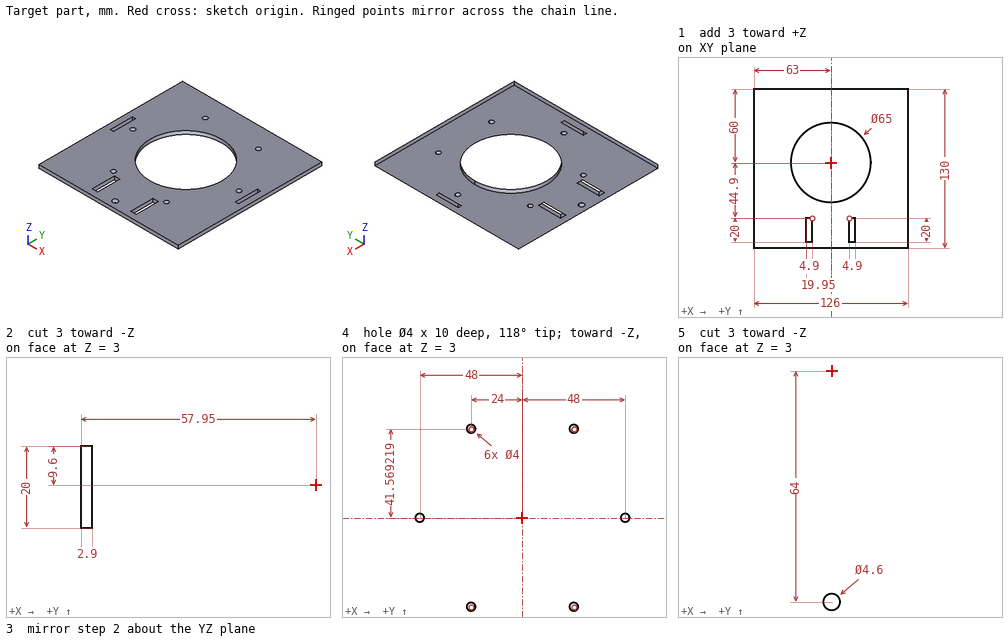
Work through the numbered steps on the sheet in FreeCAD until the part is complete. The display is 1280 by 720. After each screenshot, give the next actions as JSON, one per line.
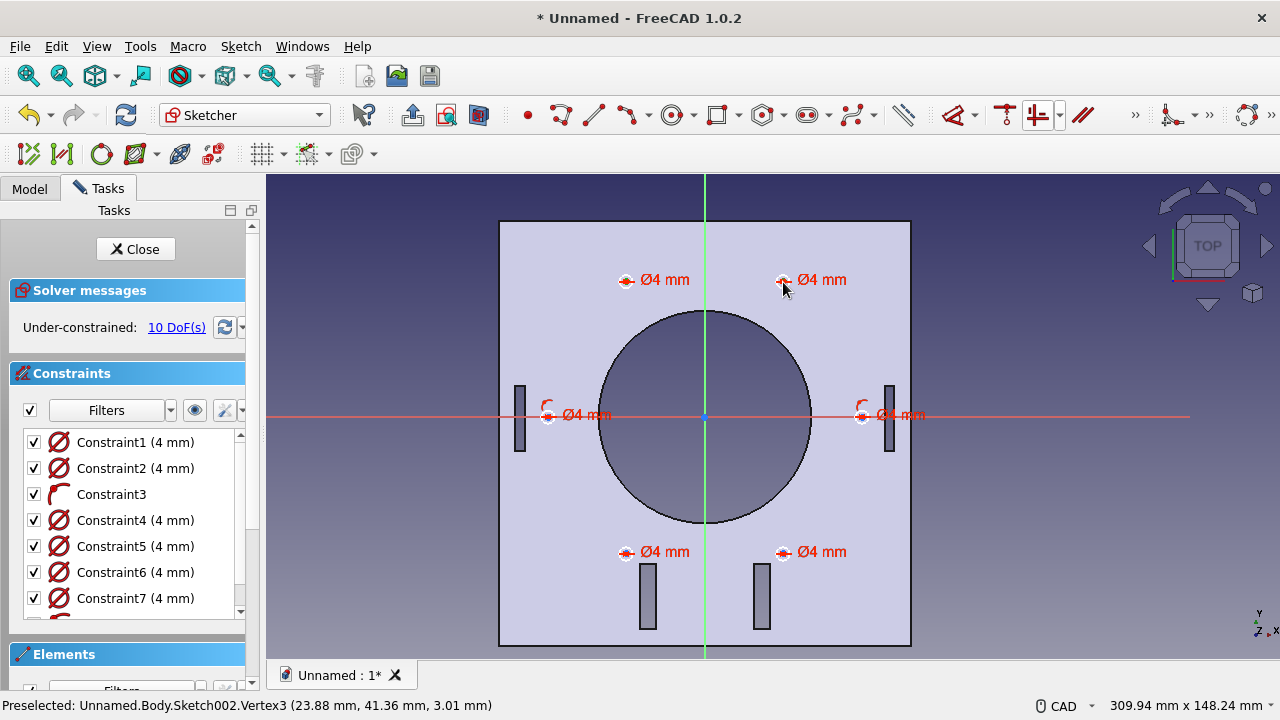
{"action": "left_click", "coordinate": [705, 600]}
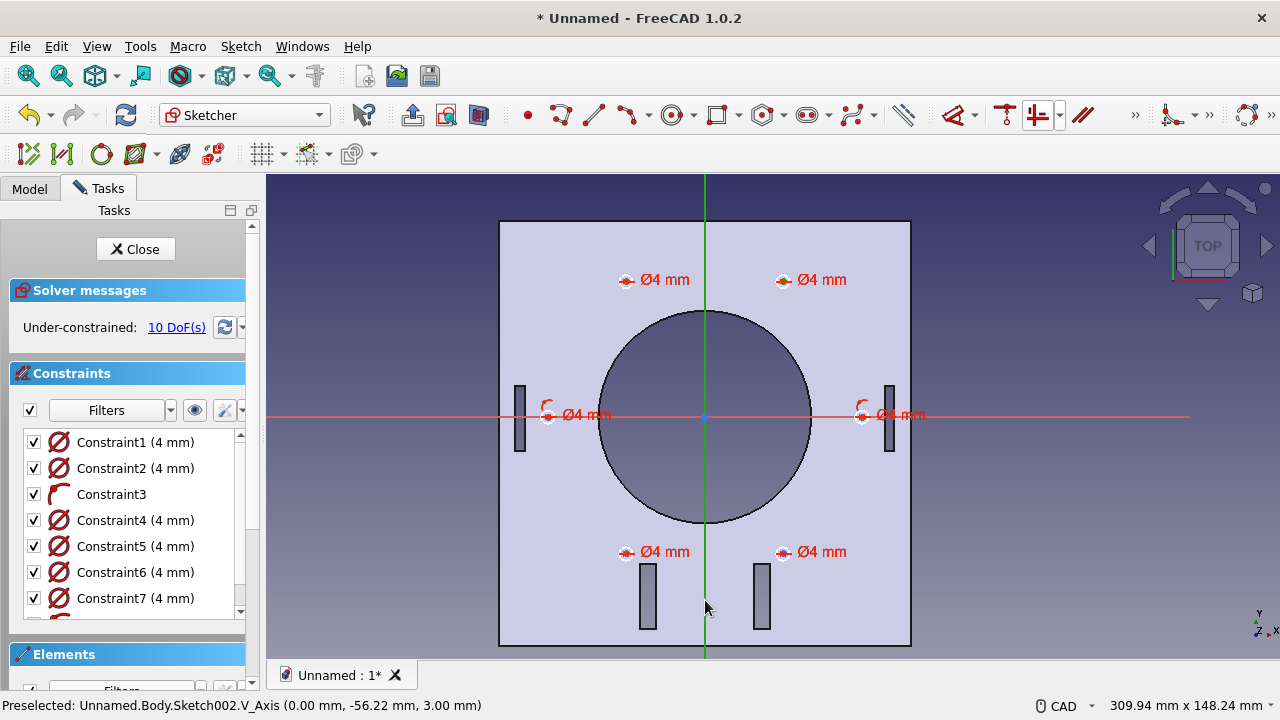
{"action": "key", "text": "s"}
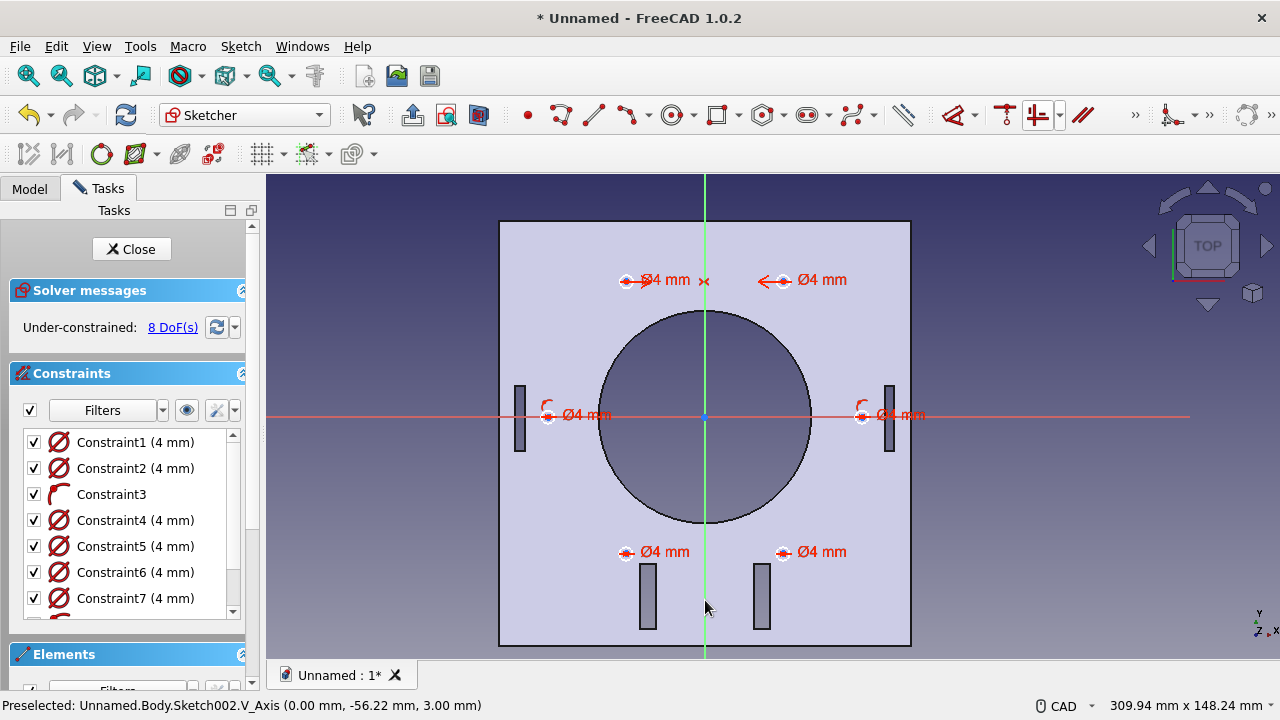
{"action": "left_click", "coordinate": [783, 282]}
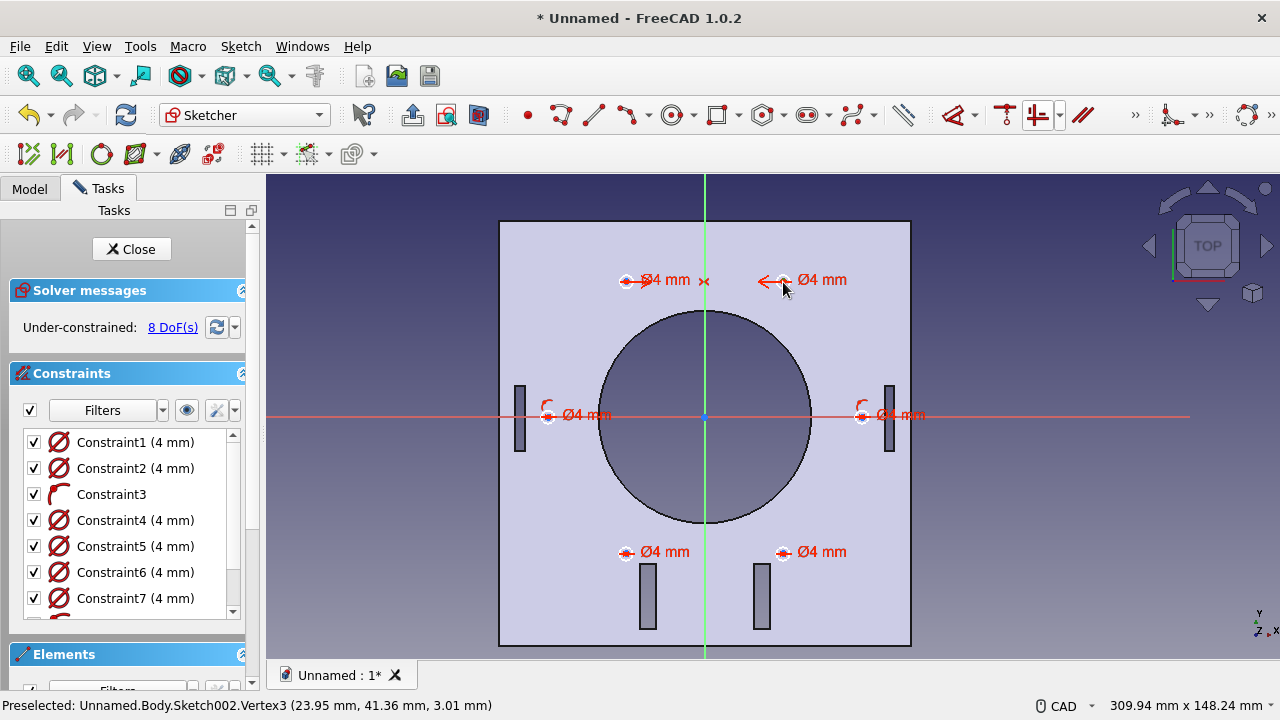
{"action": "left_click", "coordinate": [783, 554]}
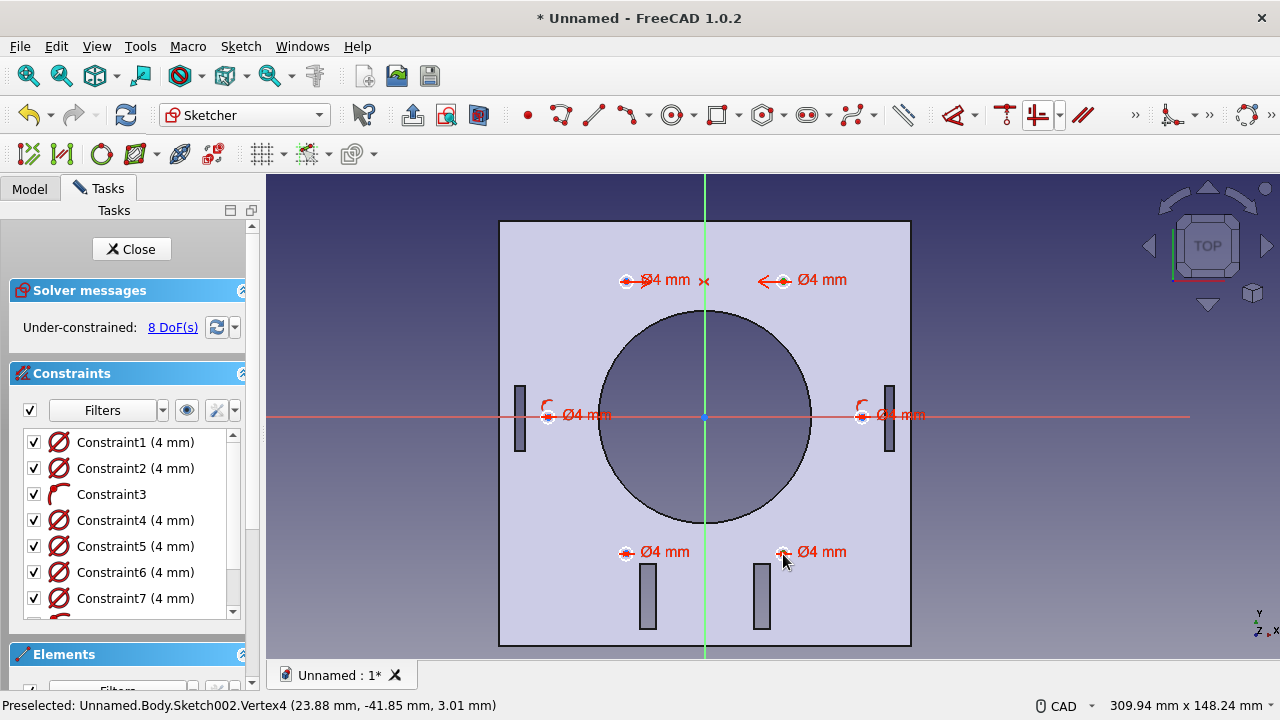
{"action": "left_click", "coordinate": [353, 417]}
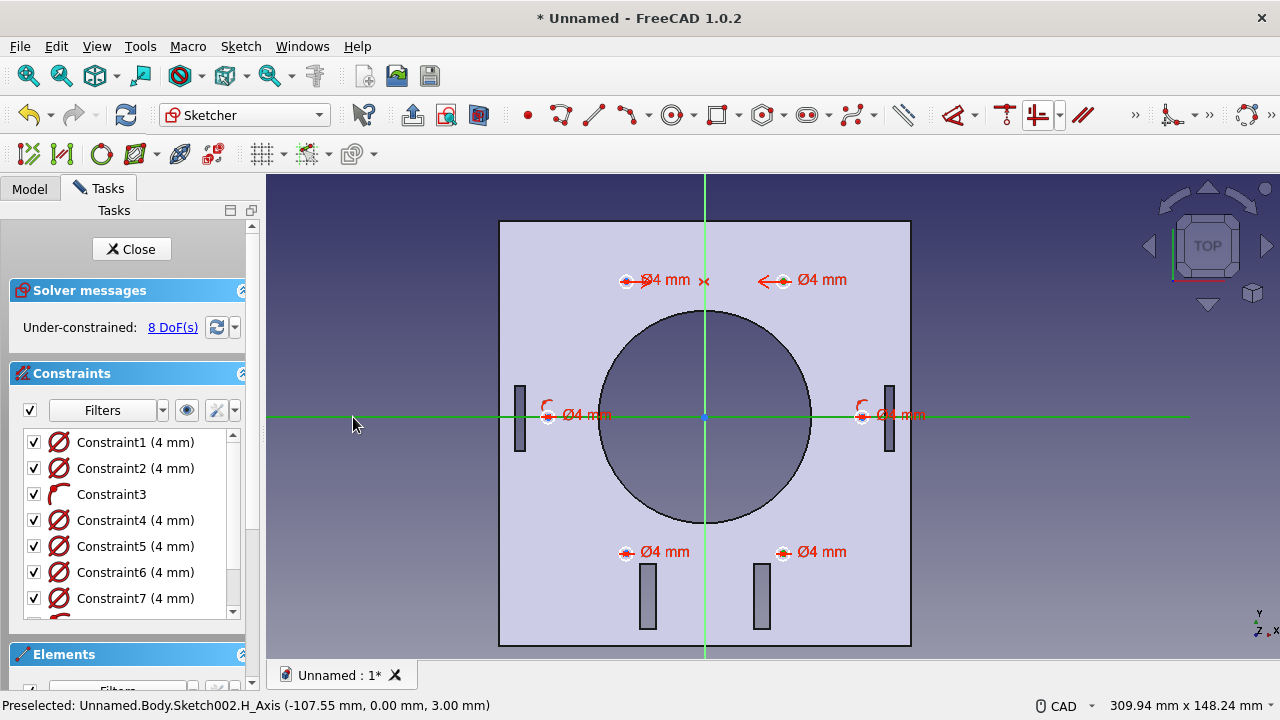
{"action": "key", "text": "s"}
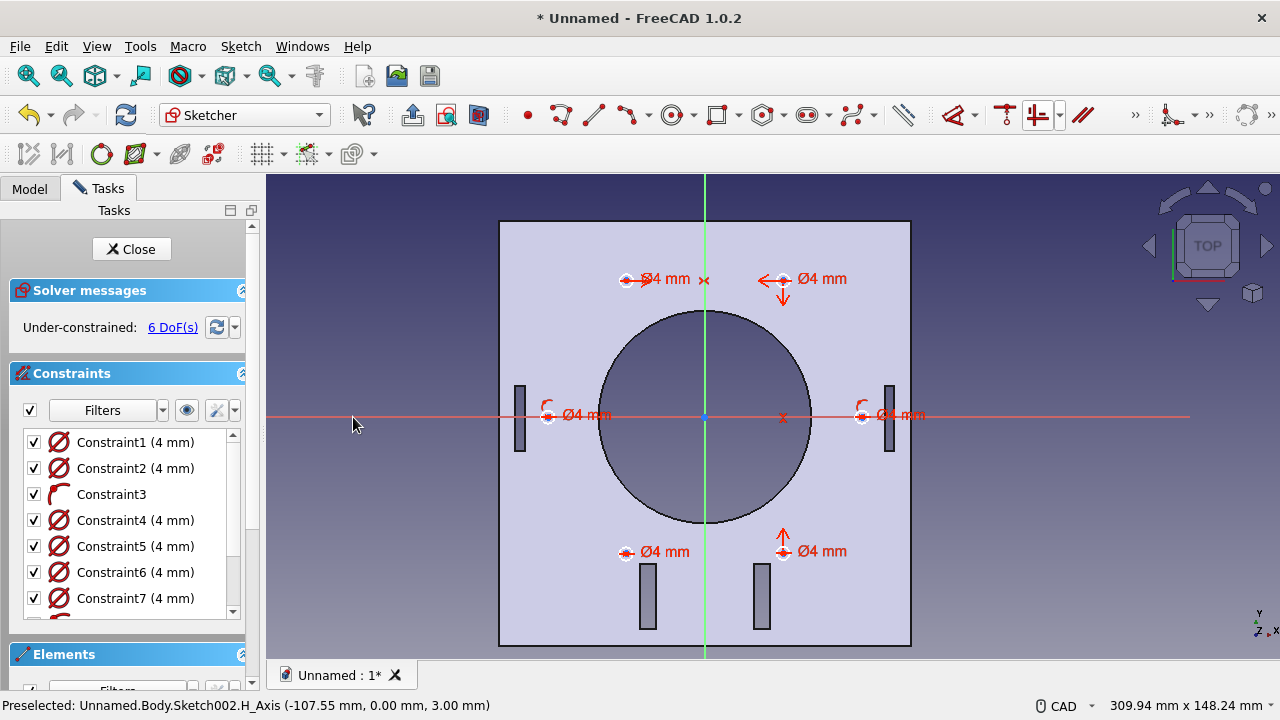
{"action": "left_click", "coordinate": [627, 281]}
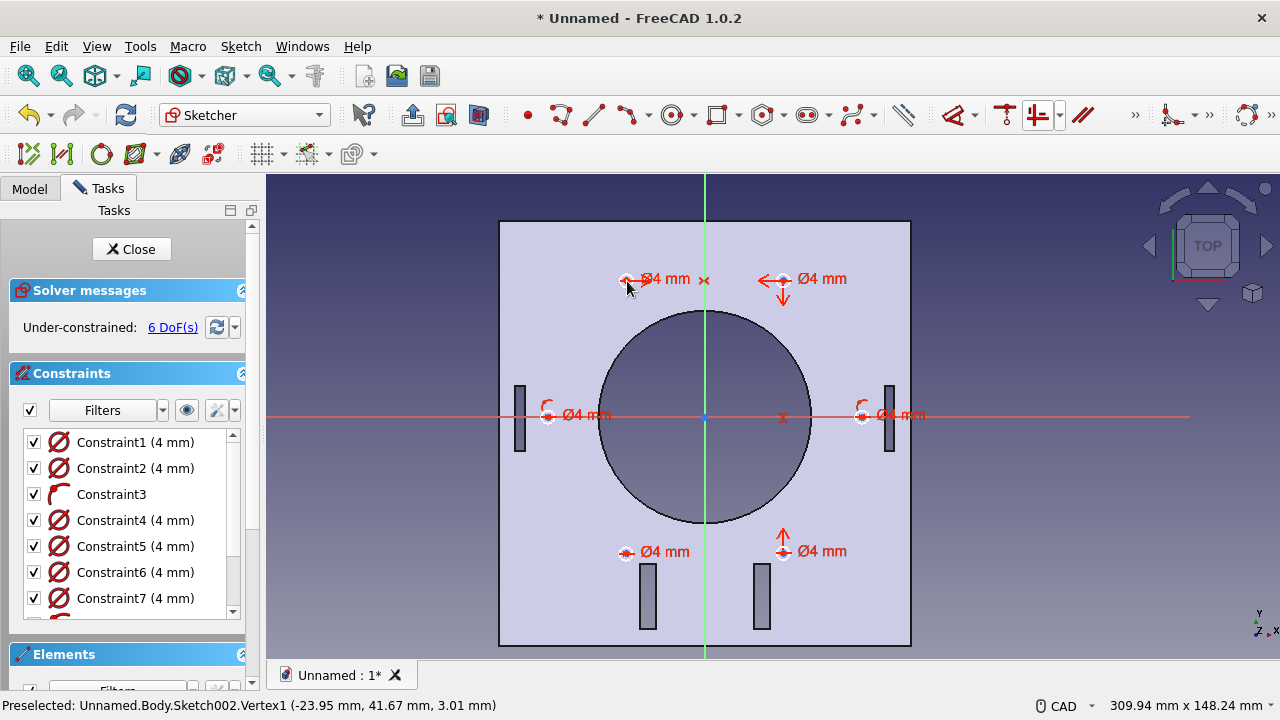
{"action": "left_click", "coordinate": [626, 554]}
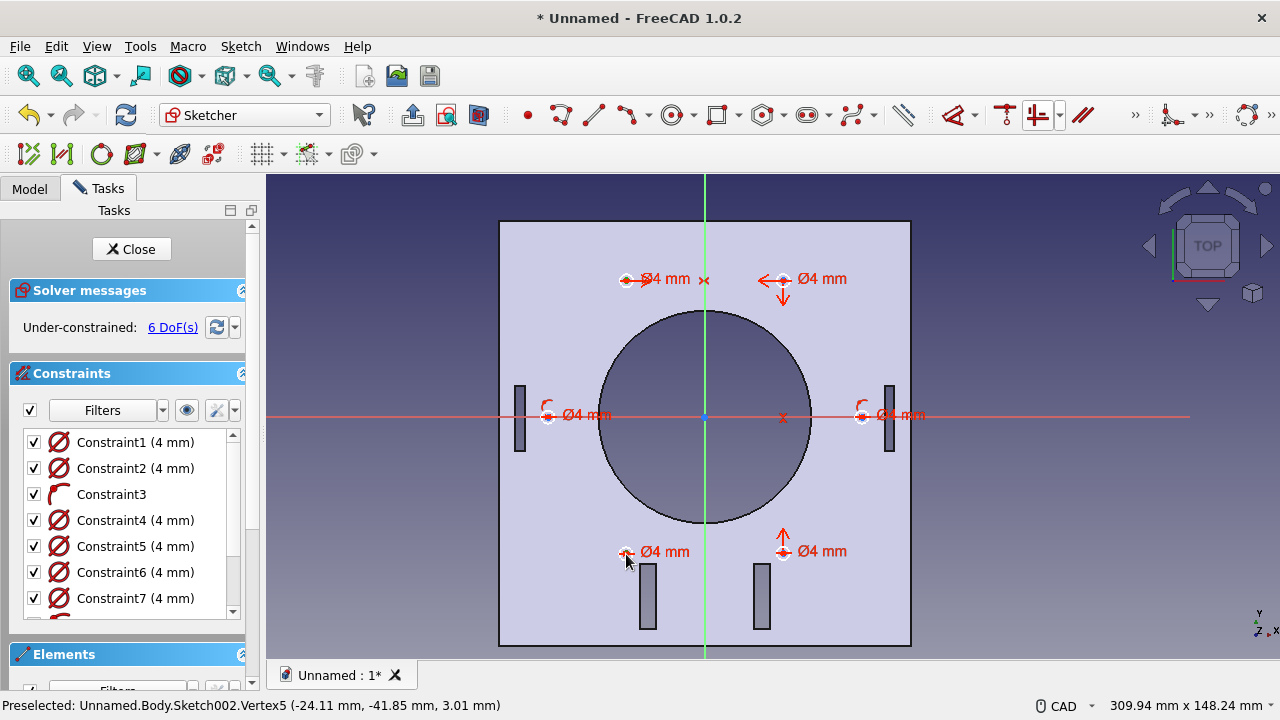
{"action": "left_click", "coordinate": [353, 417]}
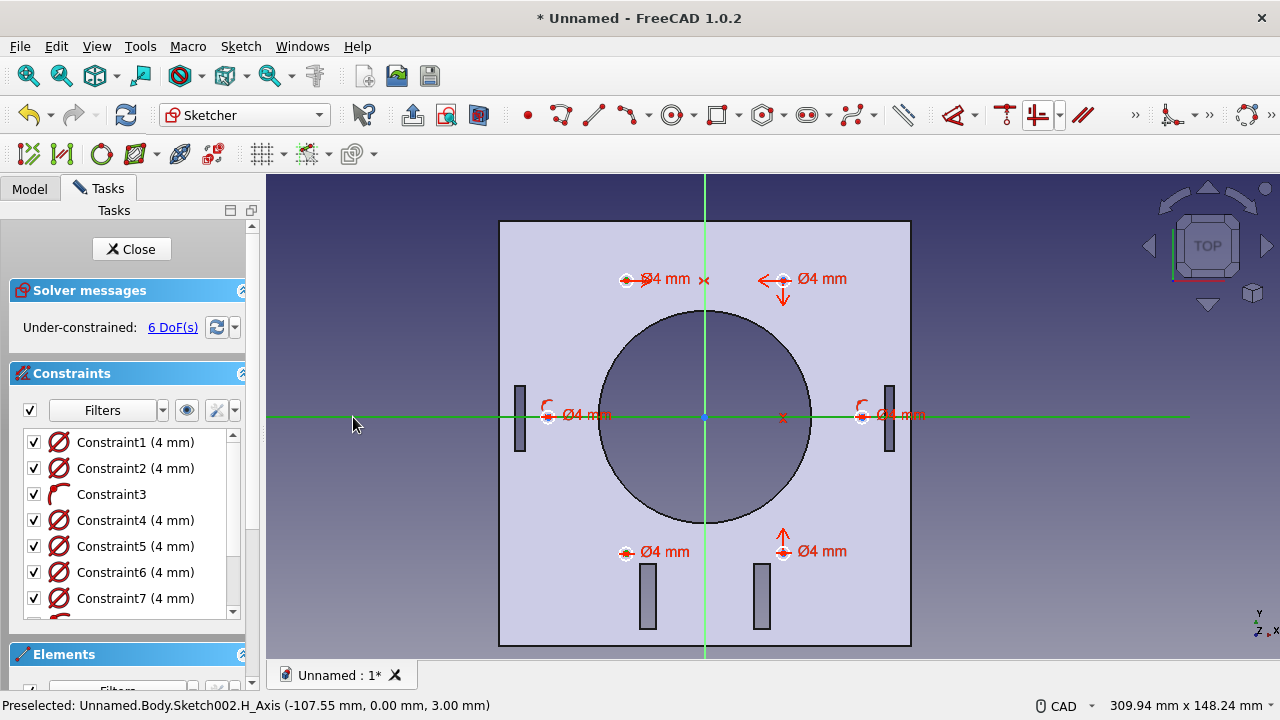
{"action": "key", "text": "s"}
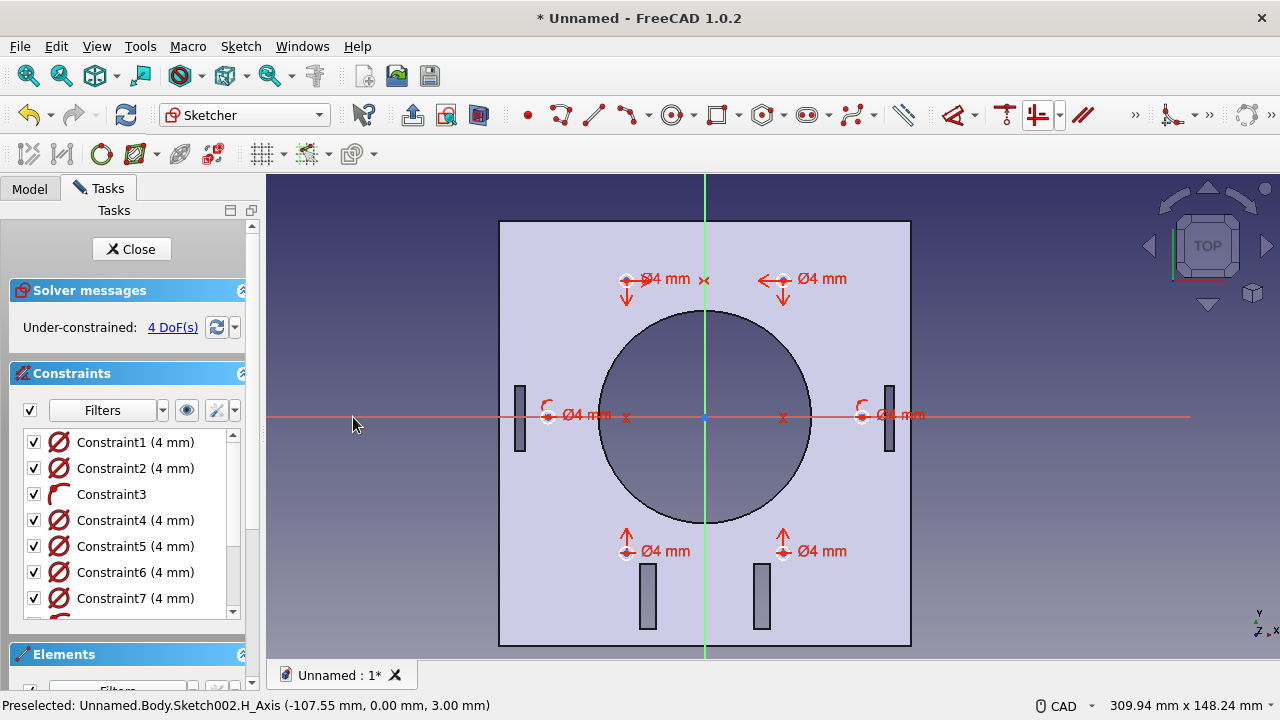
{"action": "left_click", "coordinate": [952, 116]}